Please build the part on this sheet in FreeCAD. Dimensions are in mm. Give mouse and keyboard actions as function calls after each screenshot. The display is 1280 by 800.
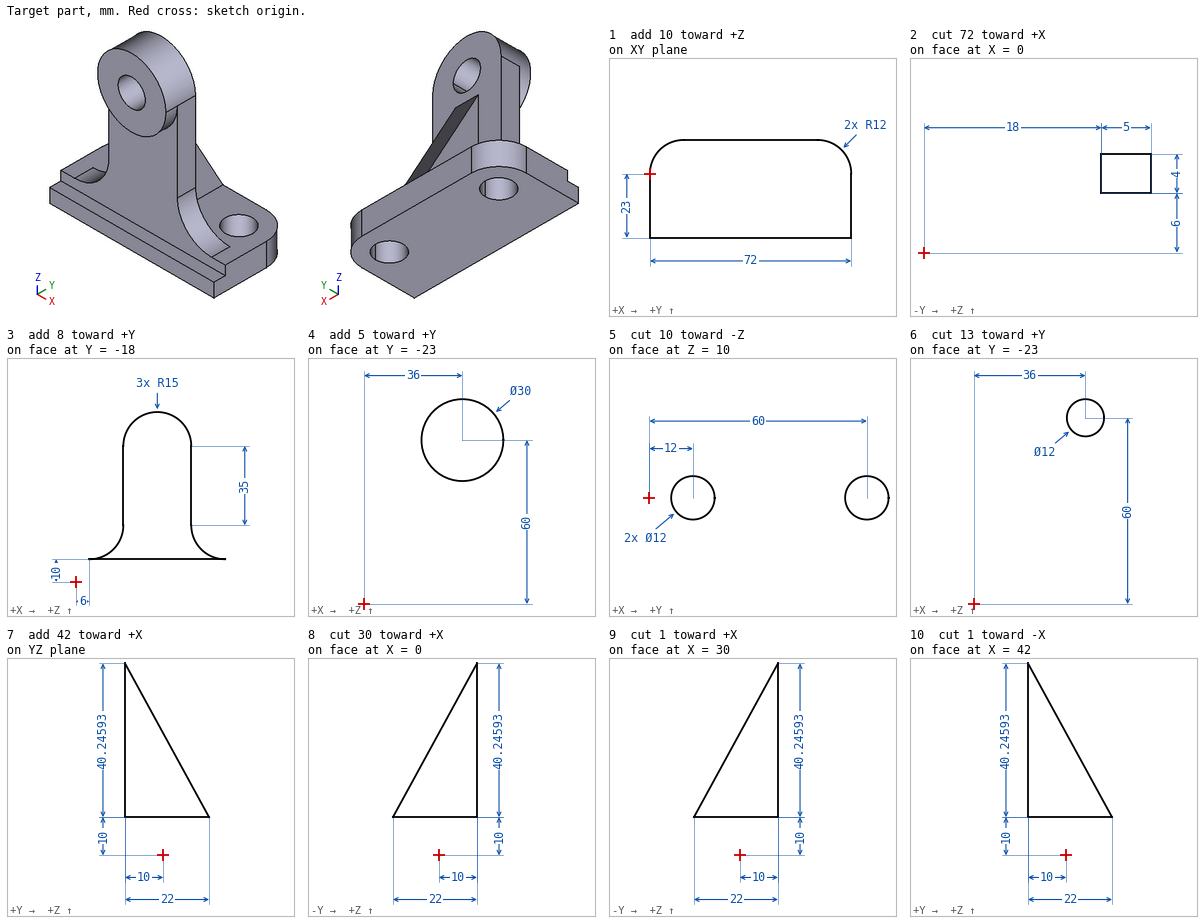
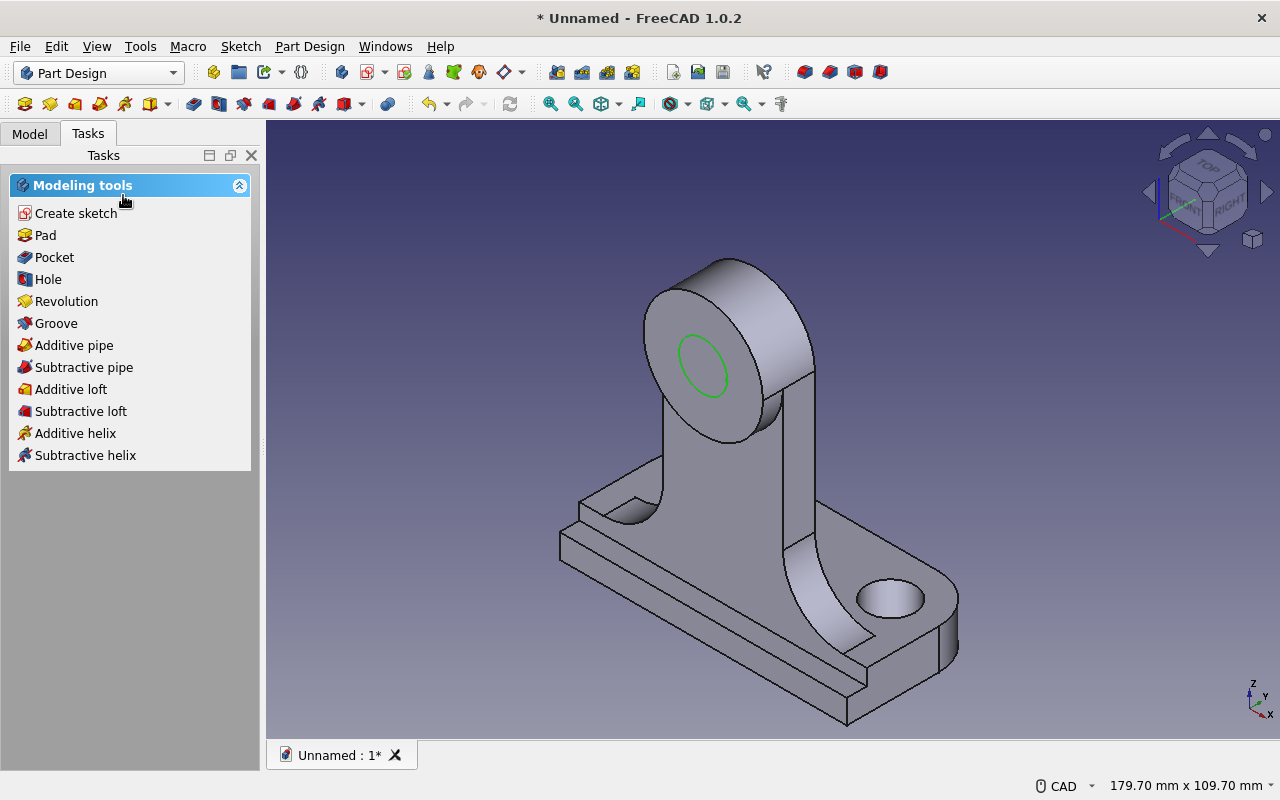
click(194, 104)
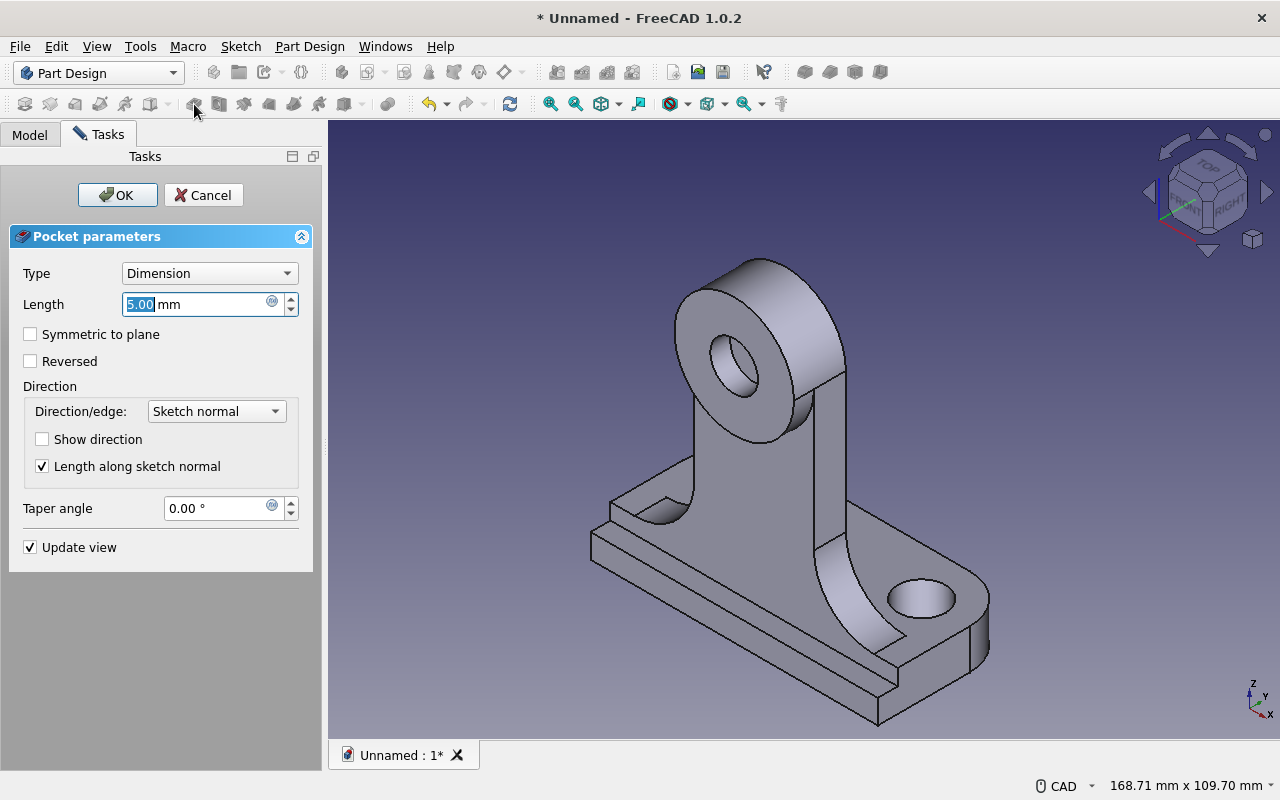
text(13)
key(Tab)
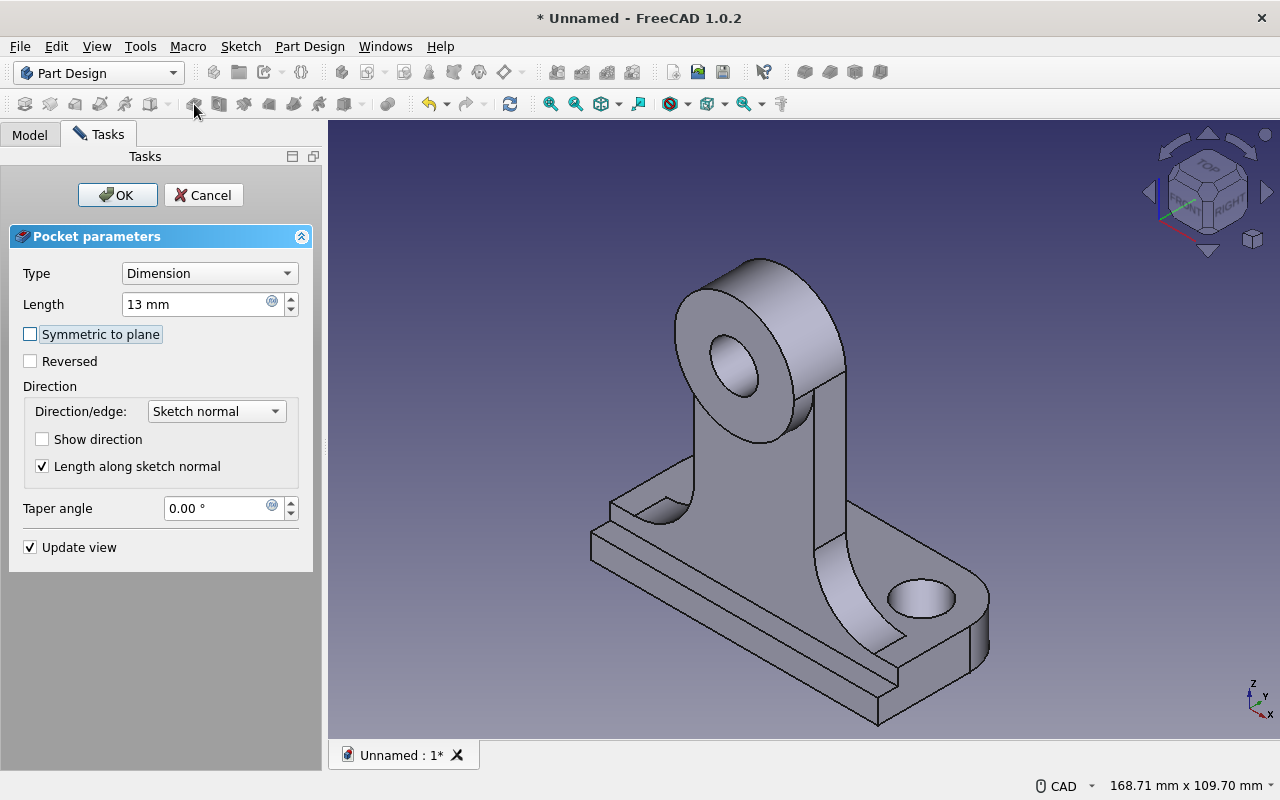
click(118, 195)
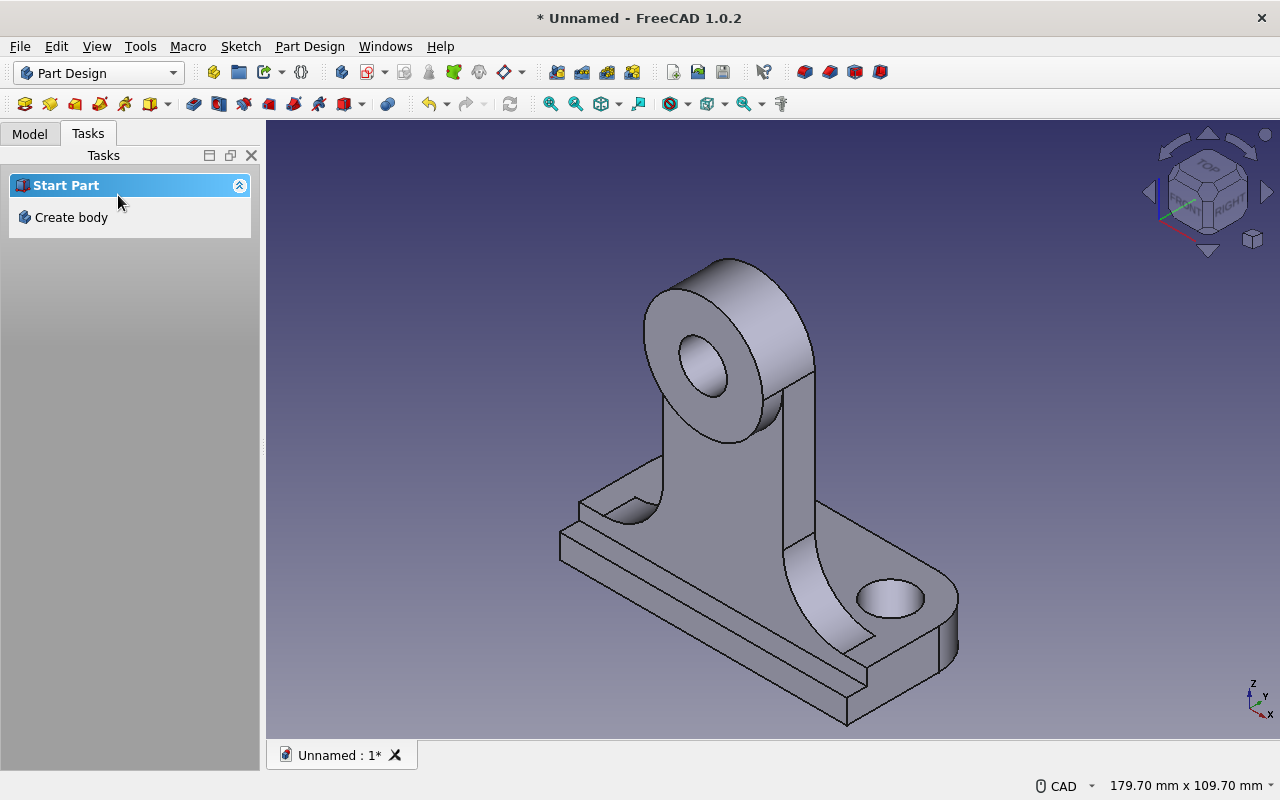
click(366, 72)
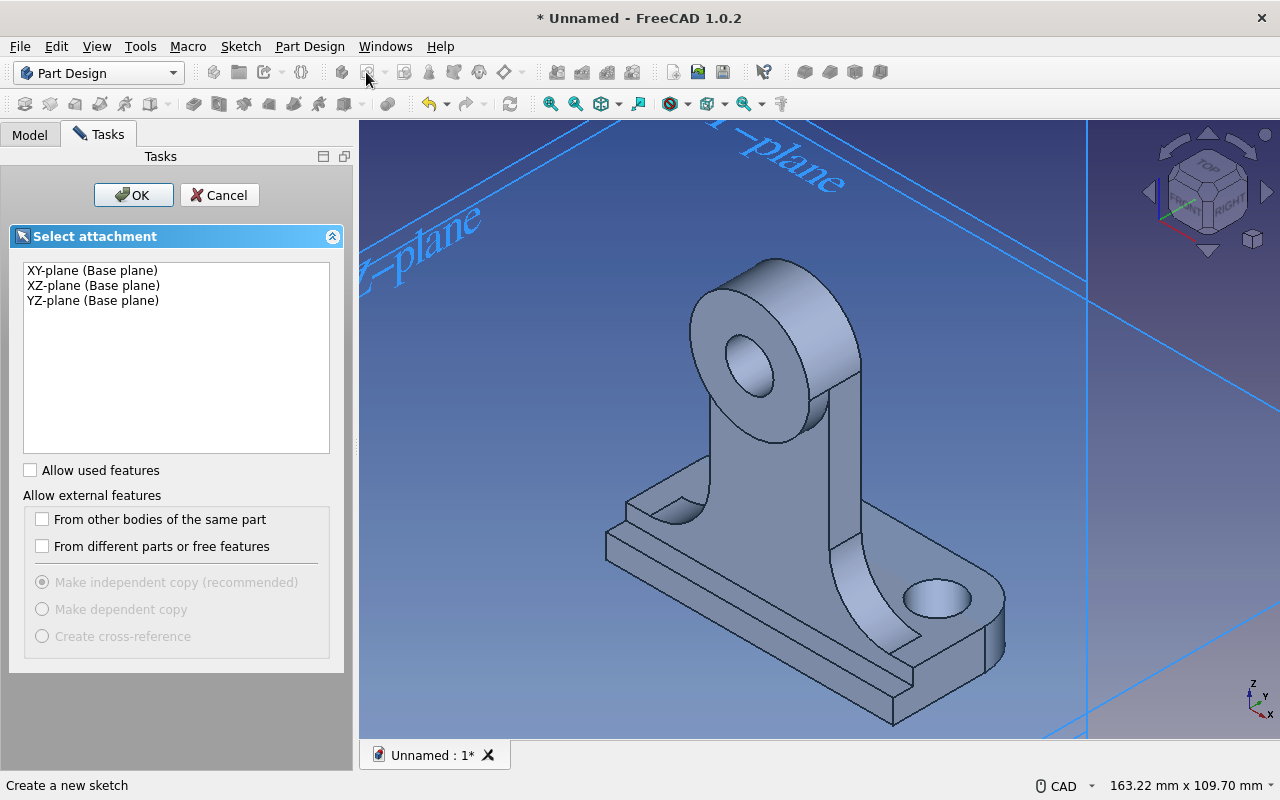
click(84, 300)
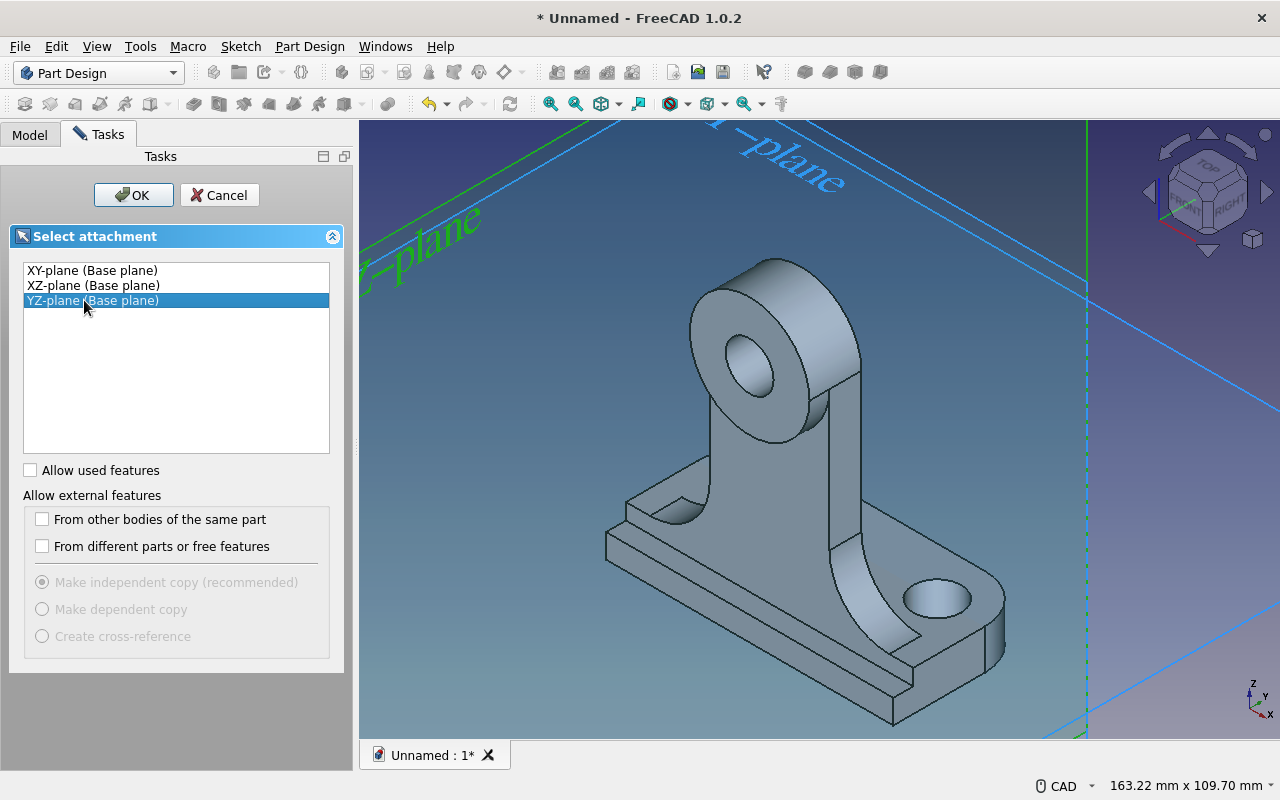
click(134, 195)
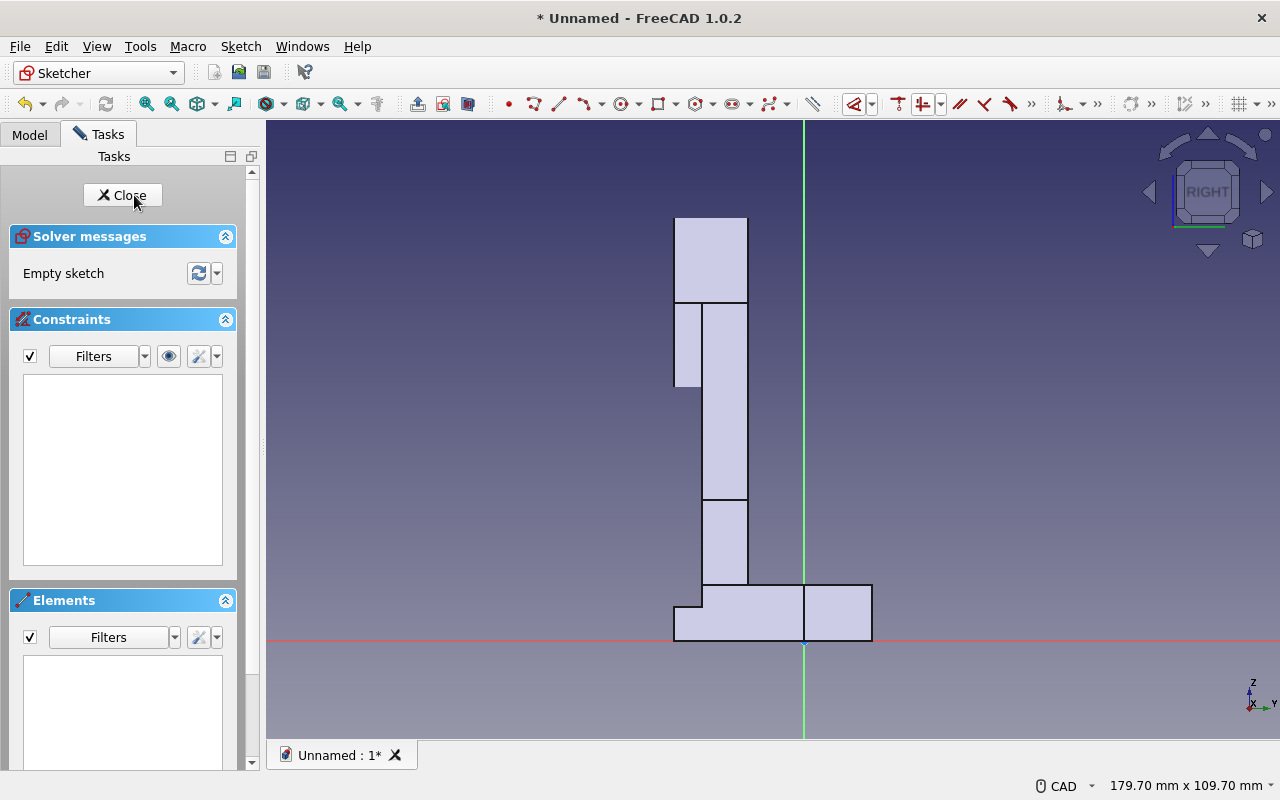
key(q)
key(s)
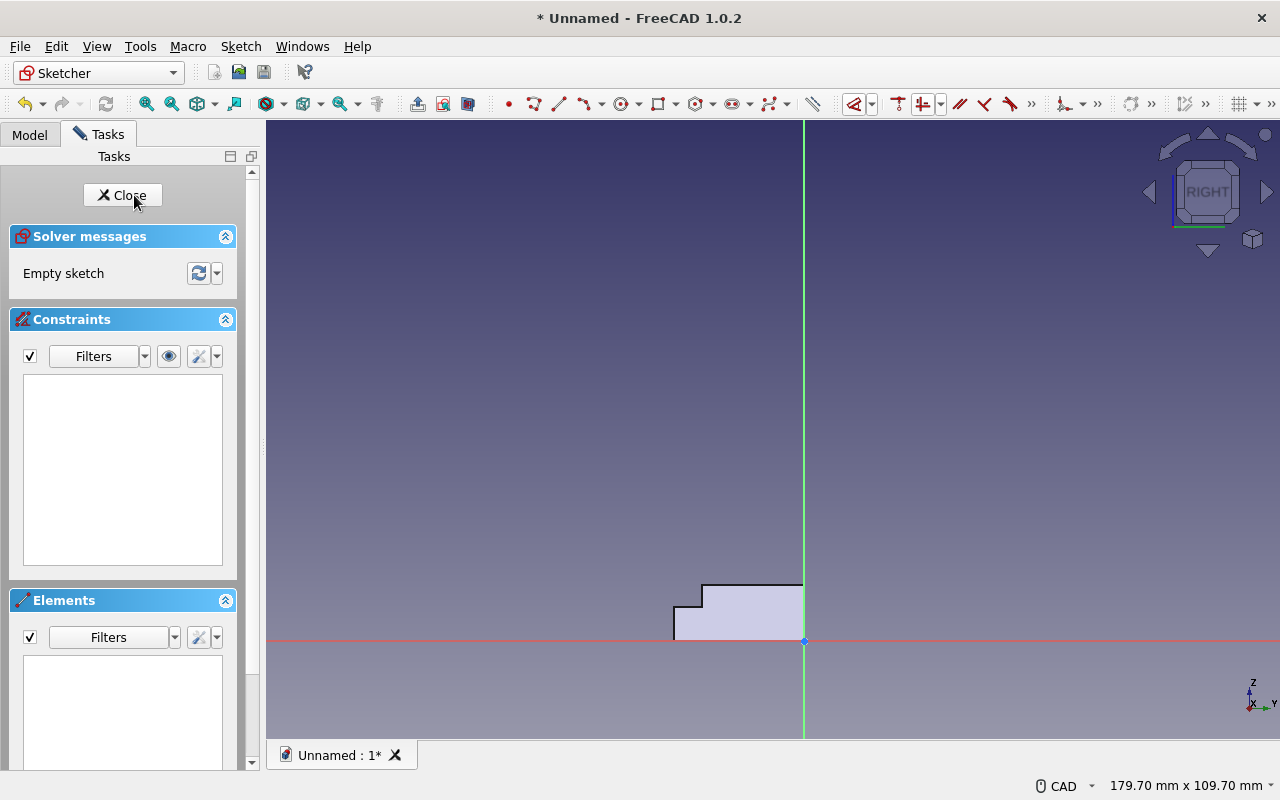
scroll(1024, 641, up, 2)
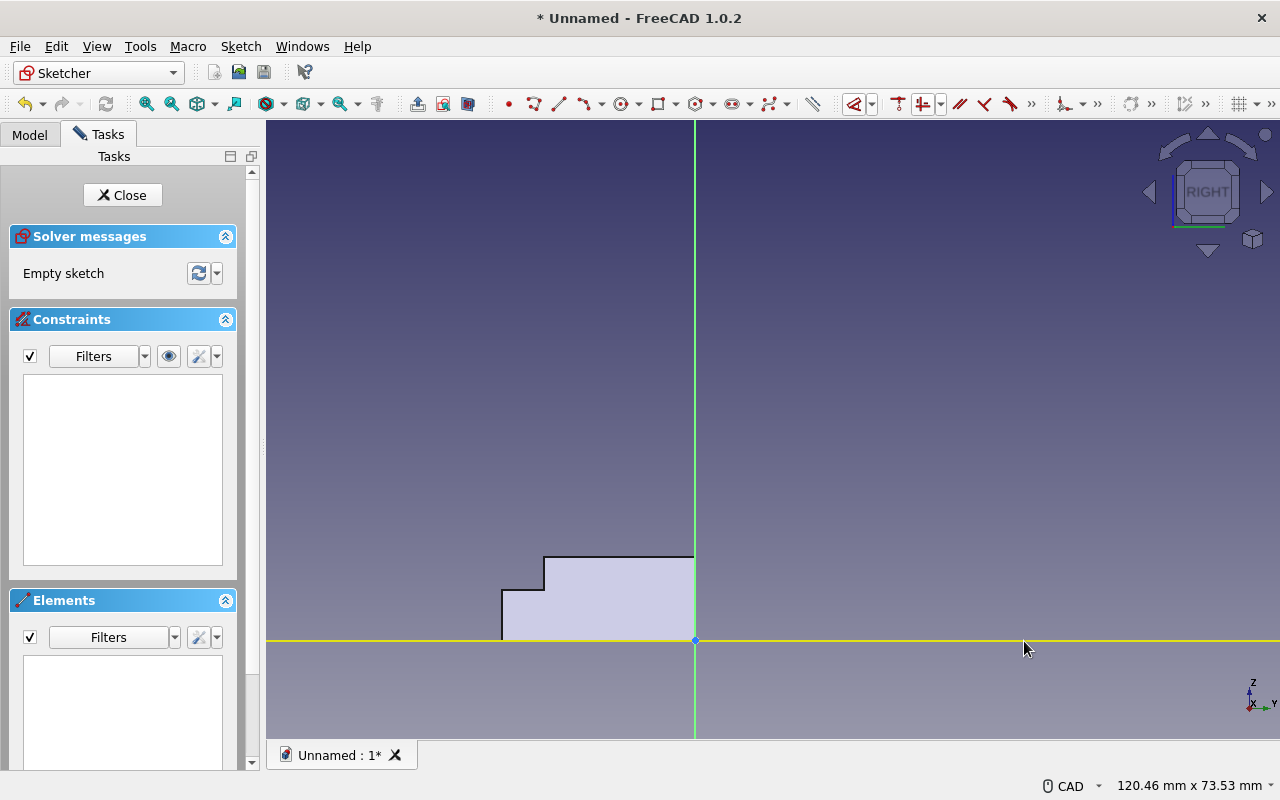
key(g)
key(m)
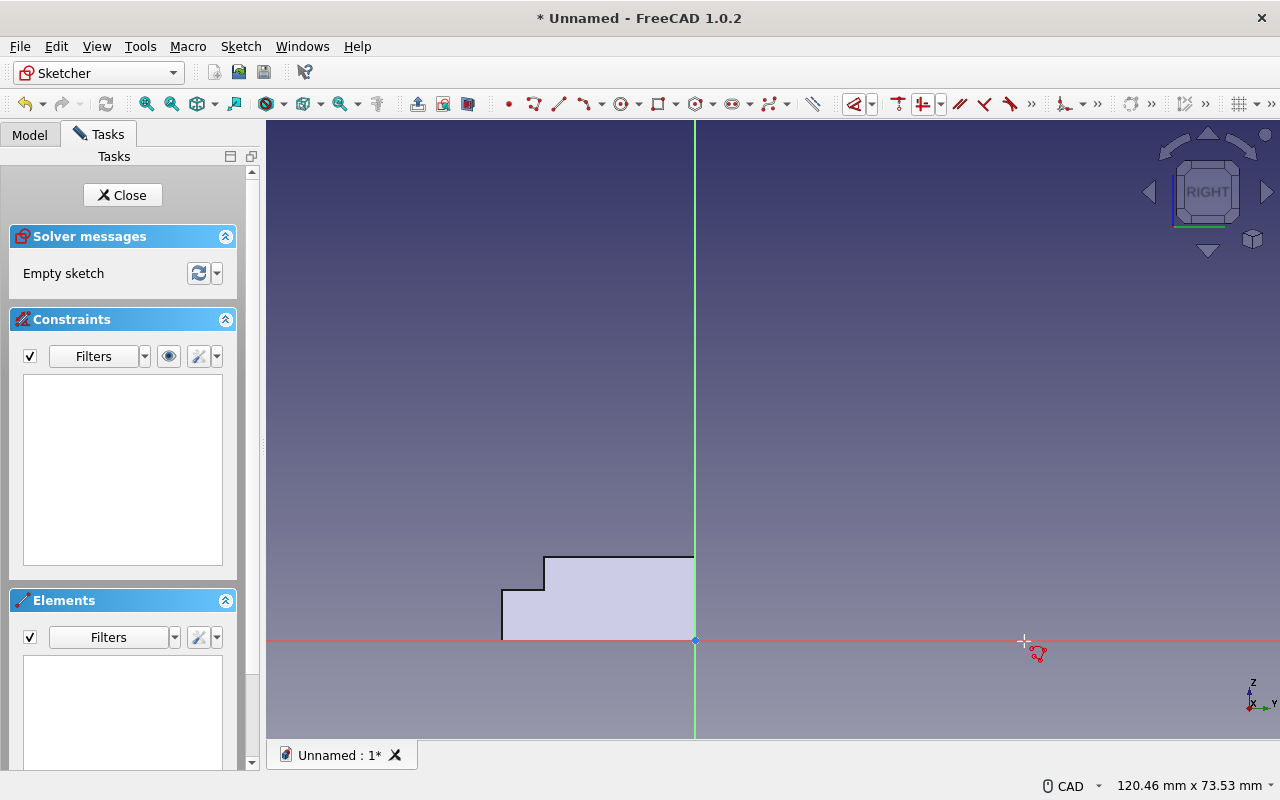
click(611, 557)
click(611, 218)
click(796, 557)
click(611, 558)
key(Escape)
key(Escape)